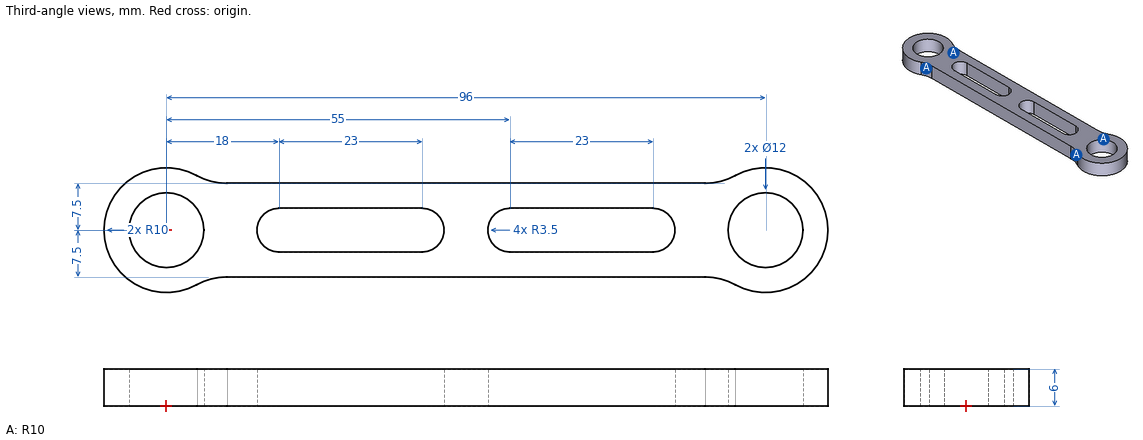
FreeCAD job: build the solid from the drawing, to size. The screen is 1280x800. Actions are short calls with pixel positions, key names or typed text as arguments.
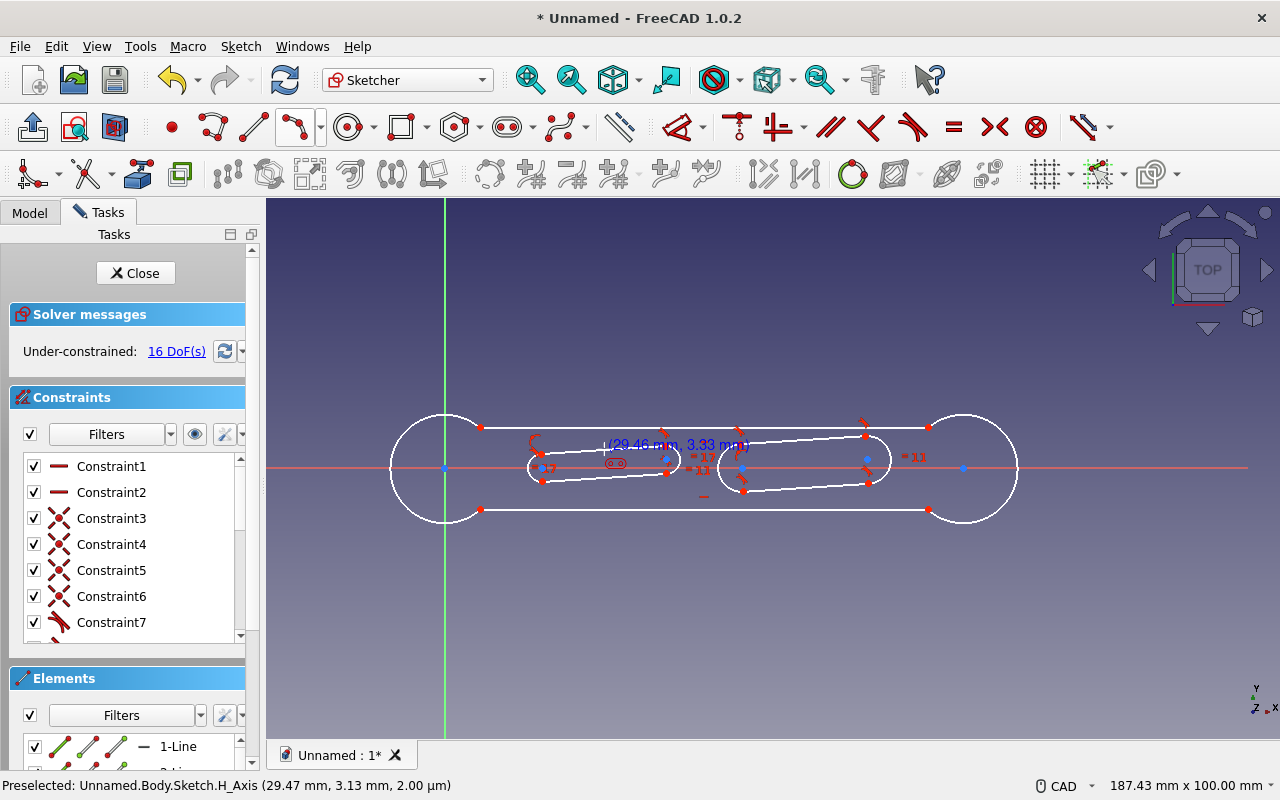
key(g)
key(c)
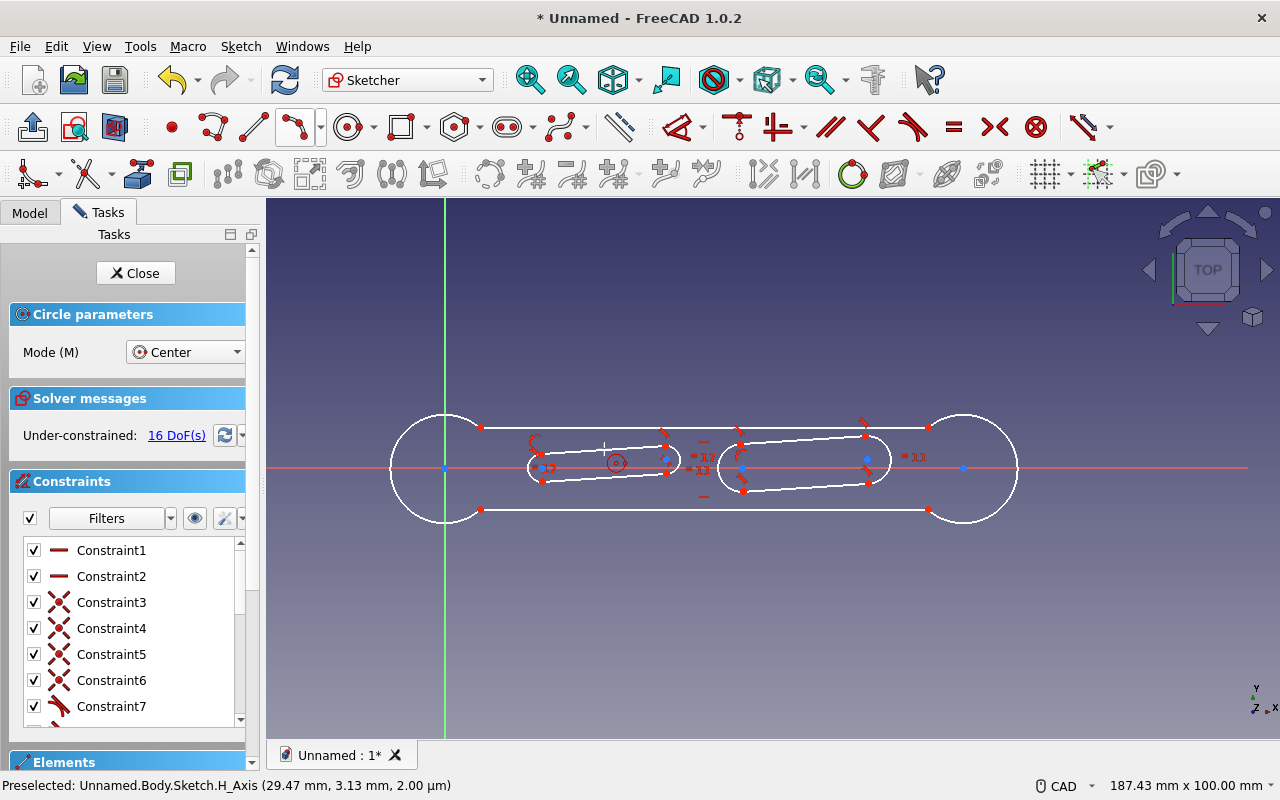
click(964, 468)
click(987, 445)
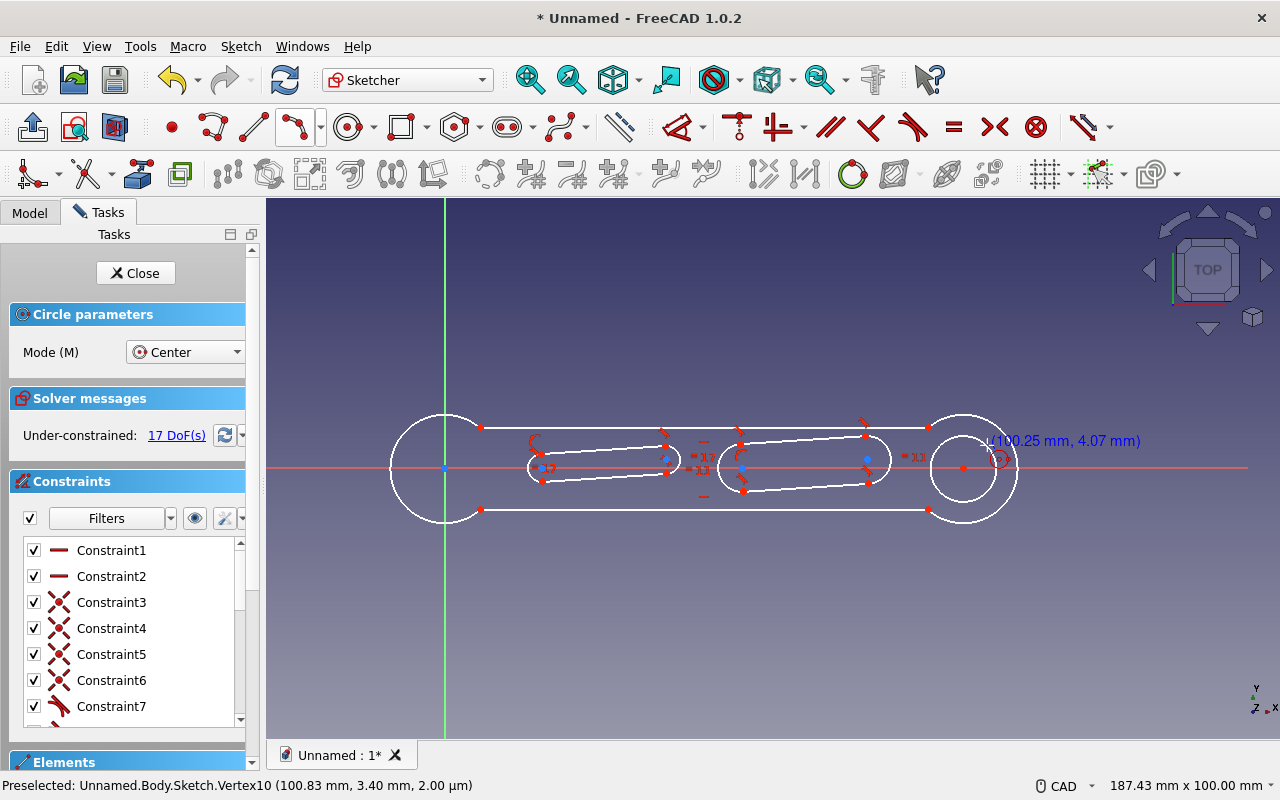
click(445, 468)
click(468, 445)
key(Escape)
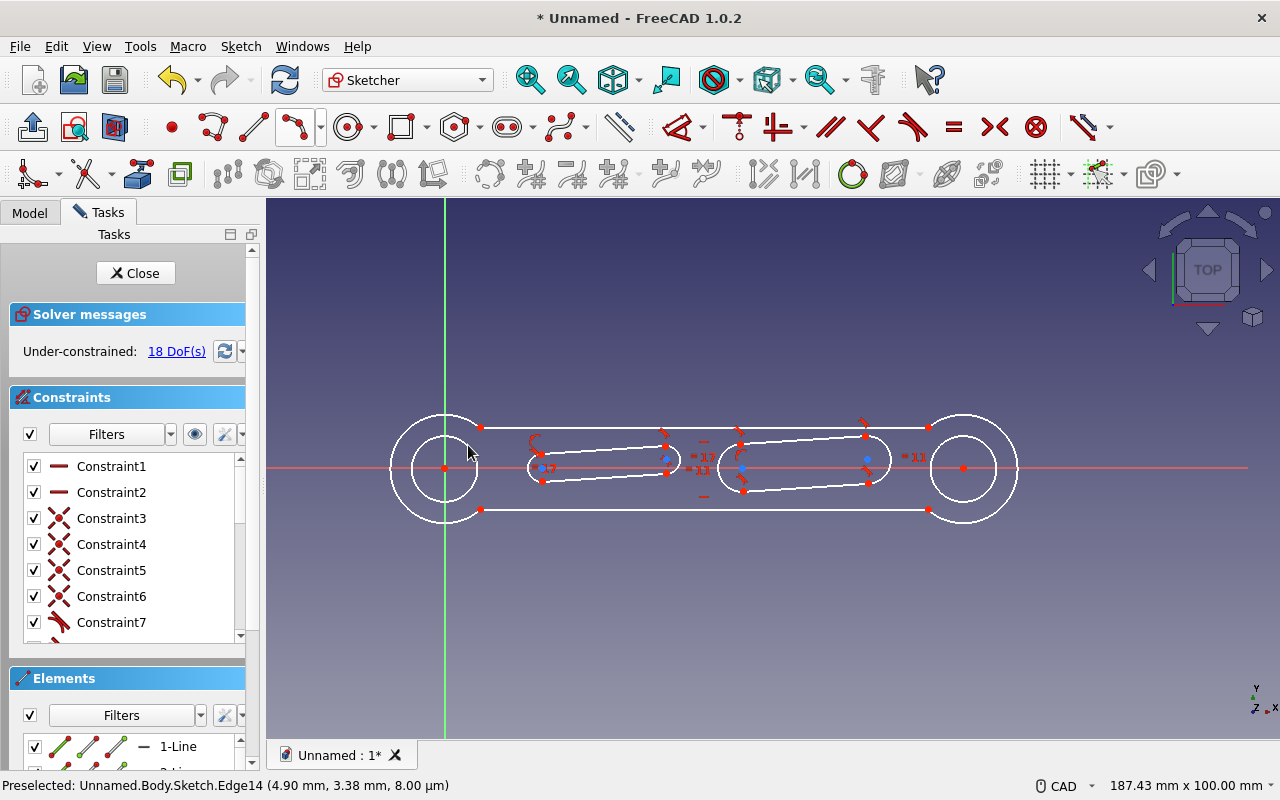
click(778, 442)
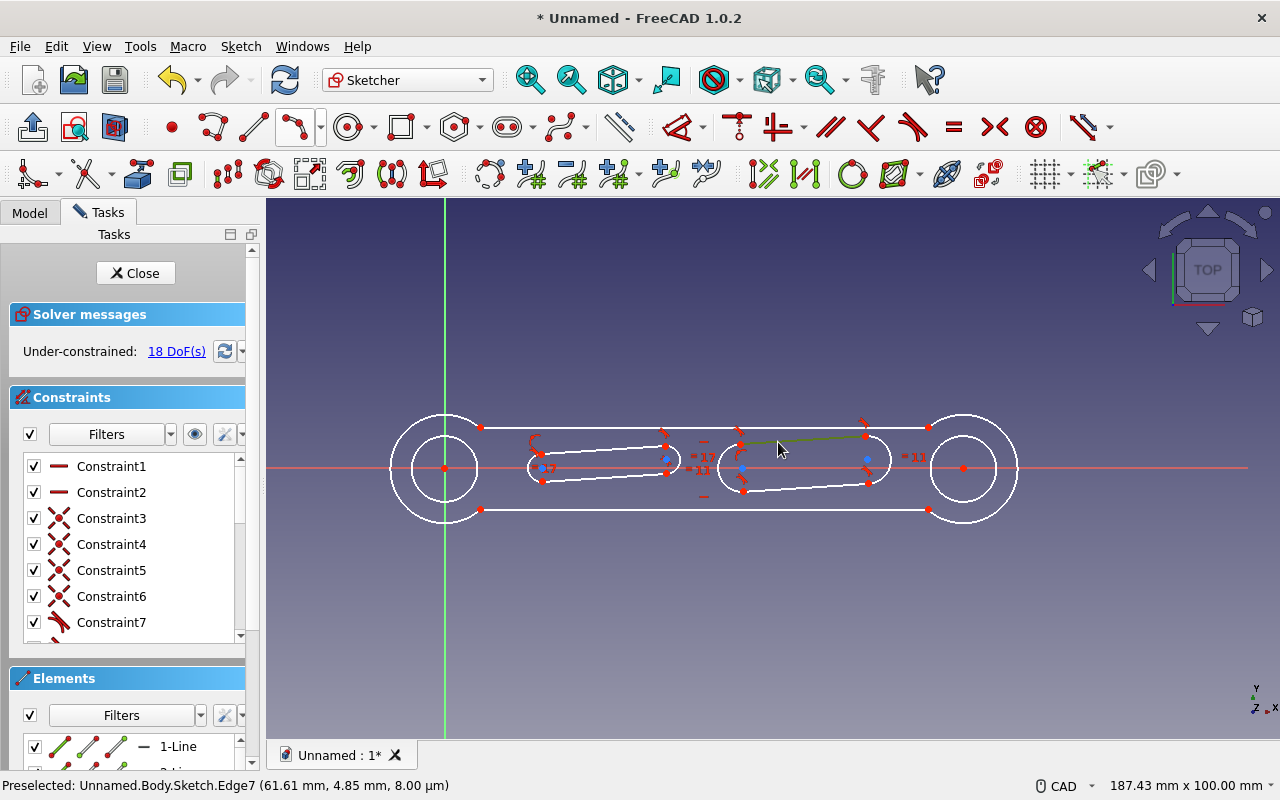
click(804, 128)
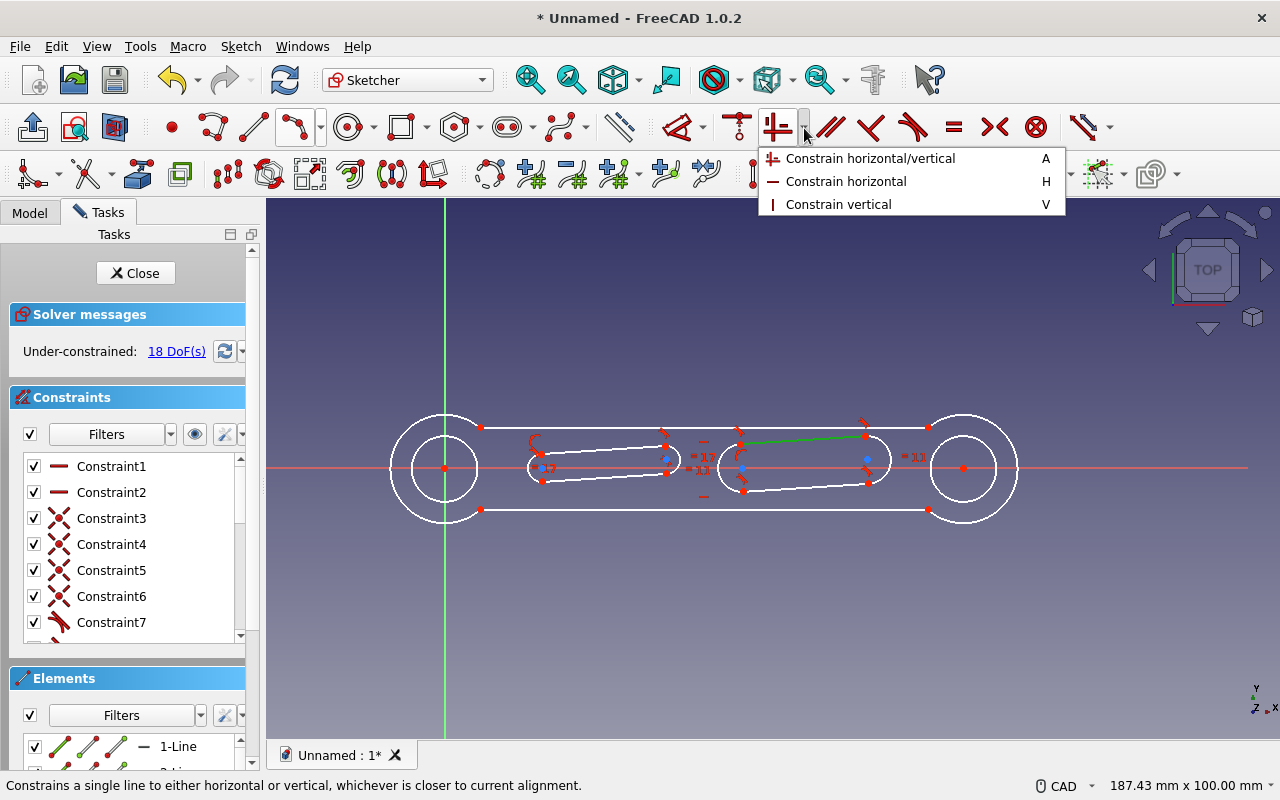
click(912, 182)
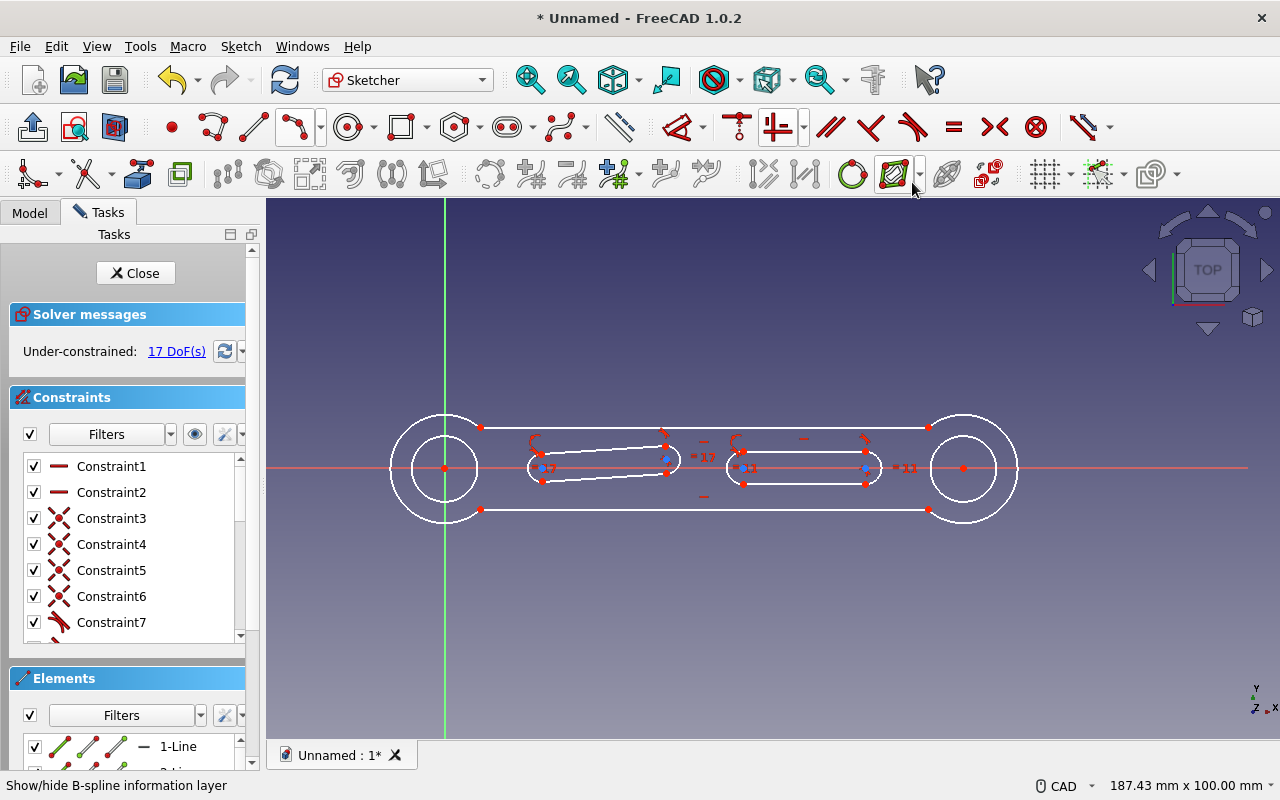
click(578, 452)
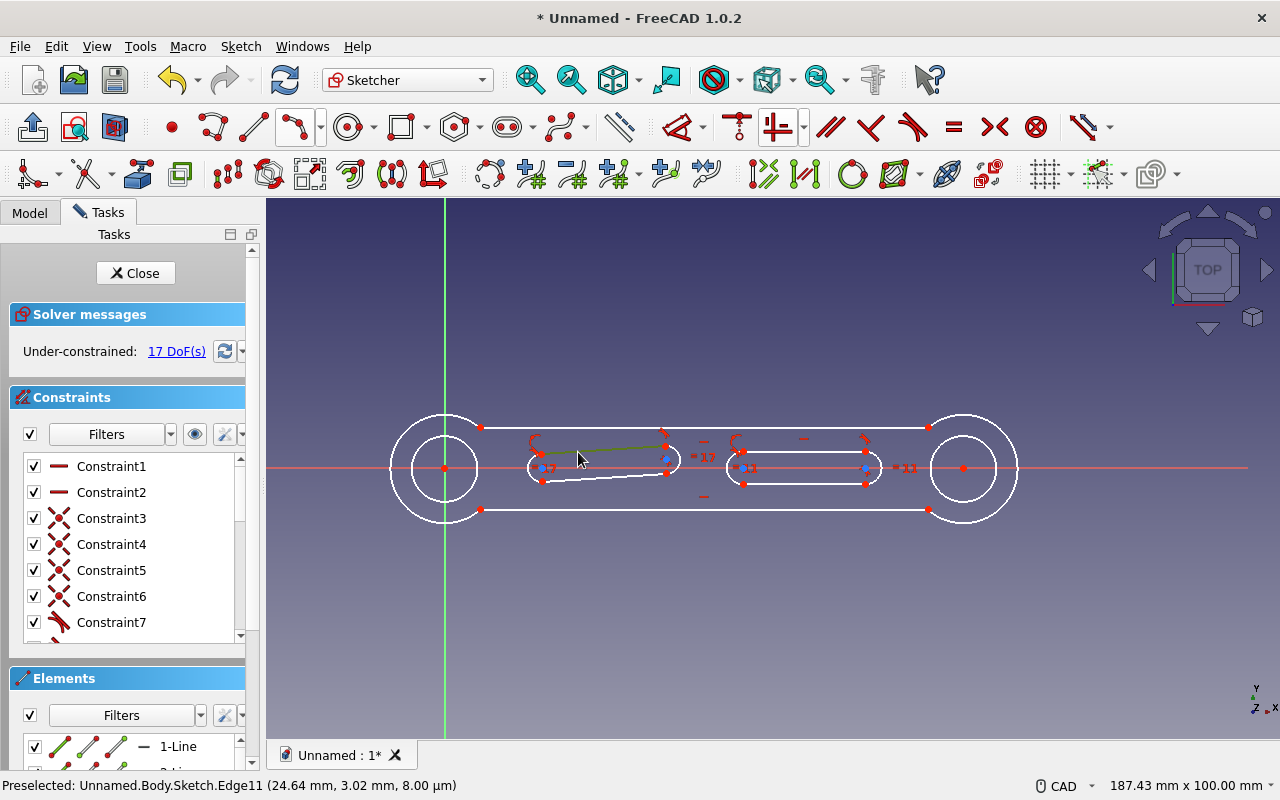
click(804, 128)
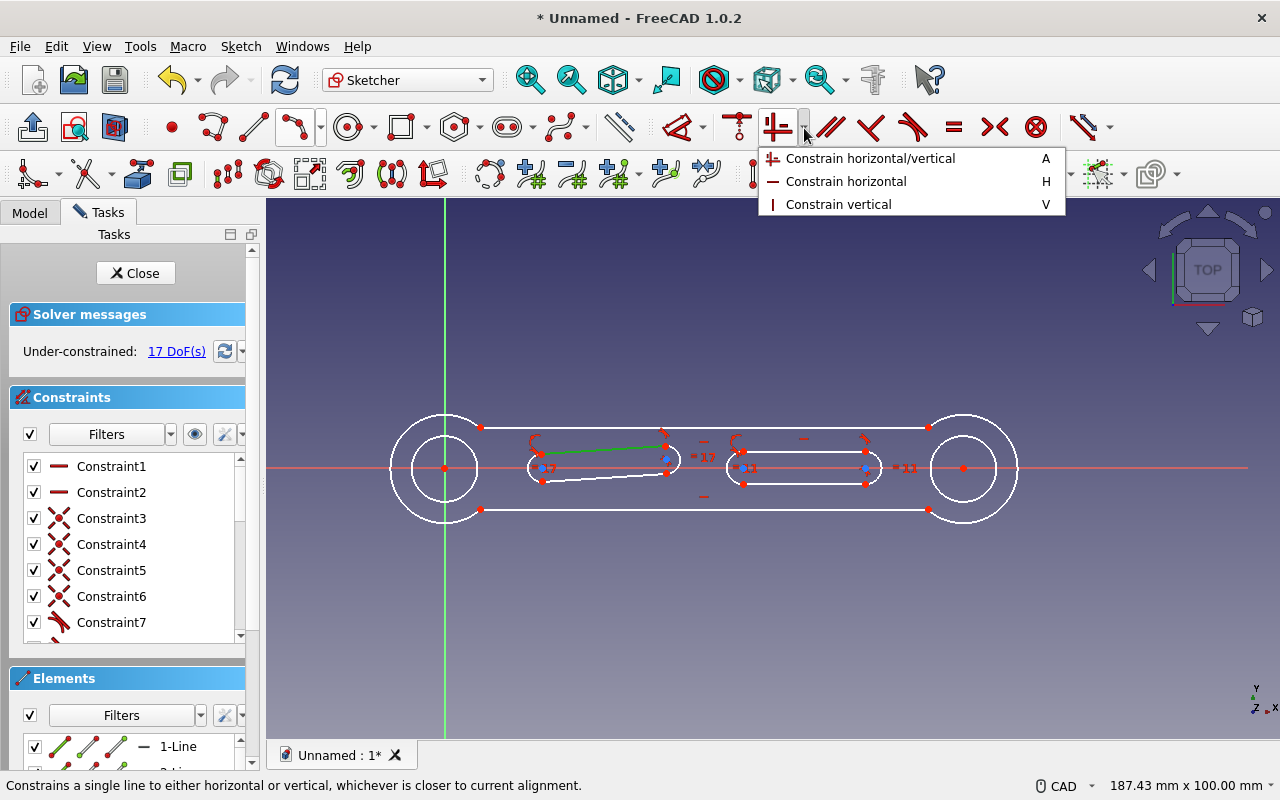
click(912, 182)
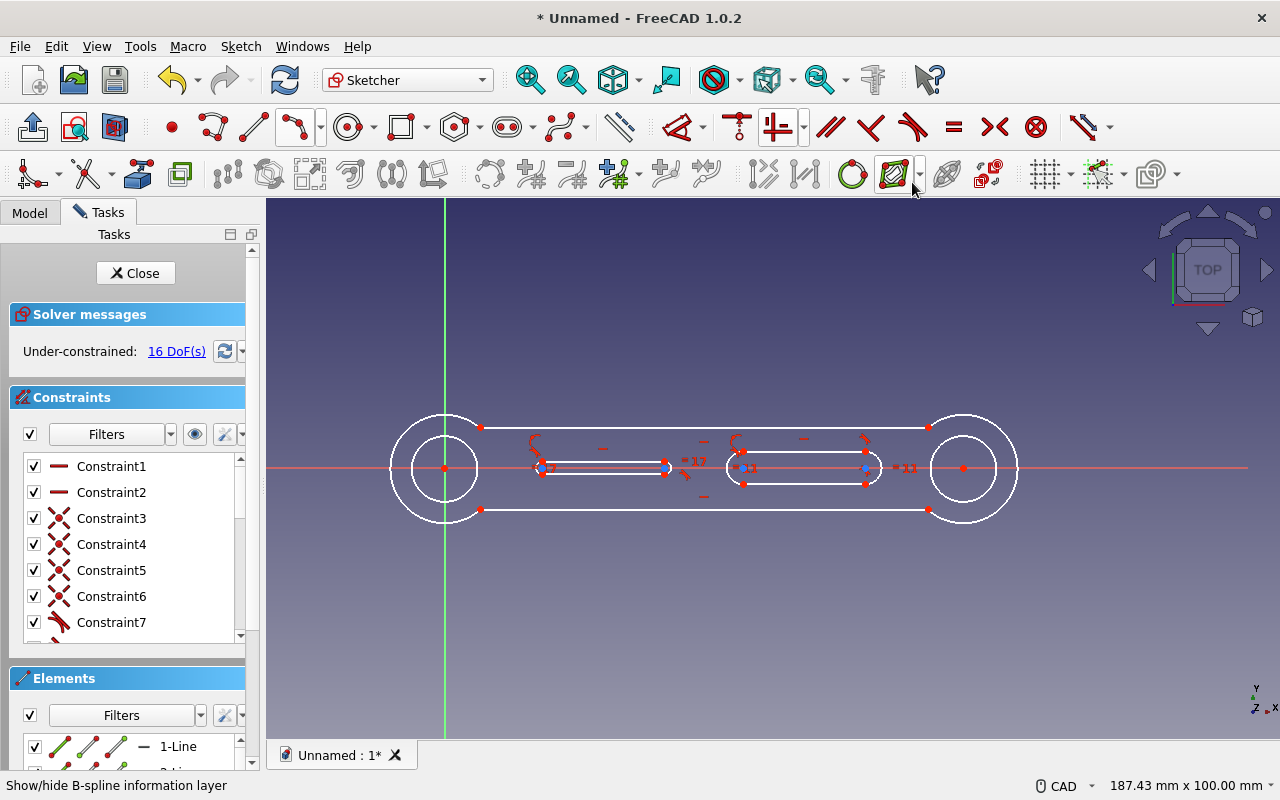
scroll(445, 469, up, 10)